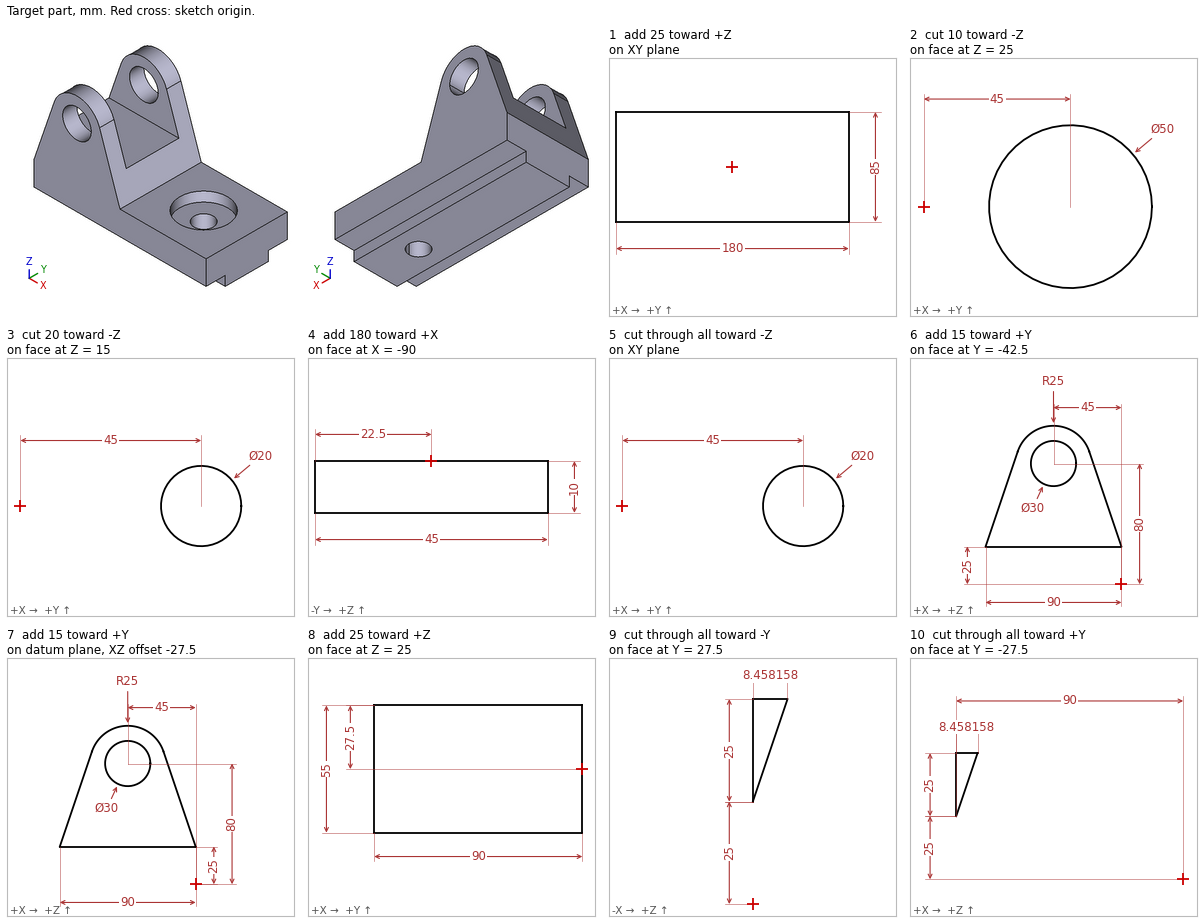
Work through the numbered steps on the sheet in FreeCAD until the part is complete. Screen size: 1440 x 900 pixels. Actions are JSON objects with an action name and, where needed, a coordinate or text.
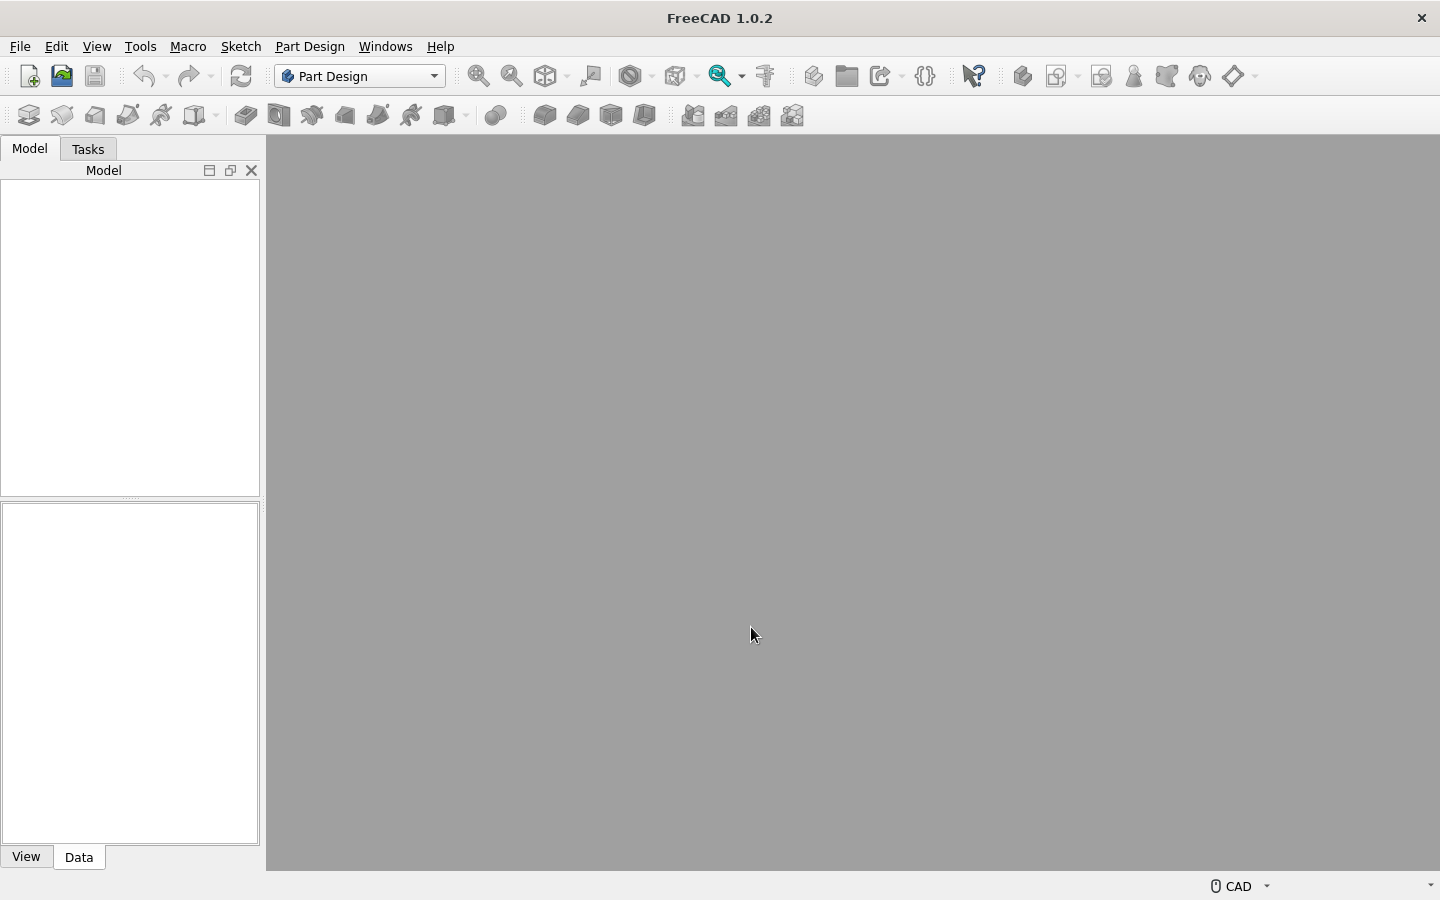
{"action": "left_click", "coordinate": [29, 76]}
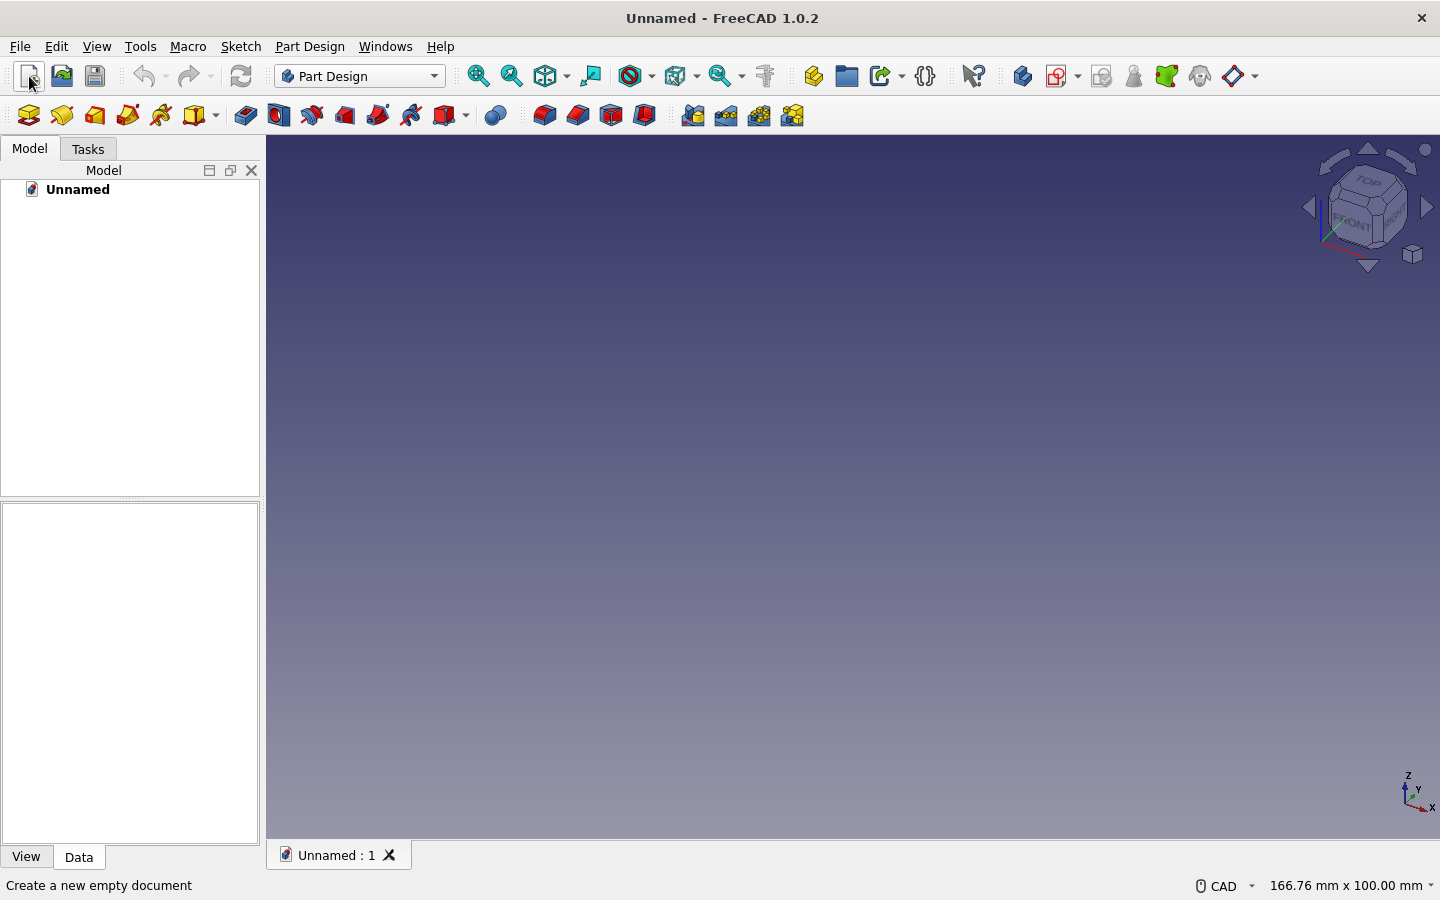
{"action": "left_click", "coordinate": [1056, 76]}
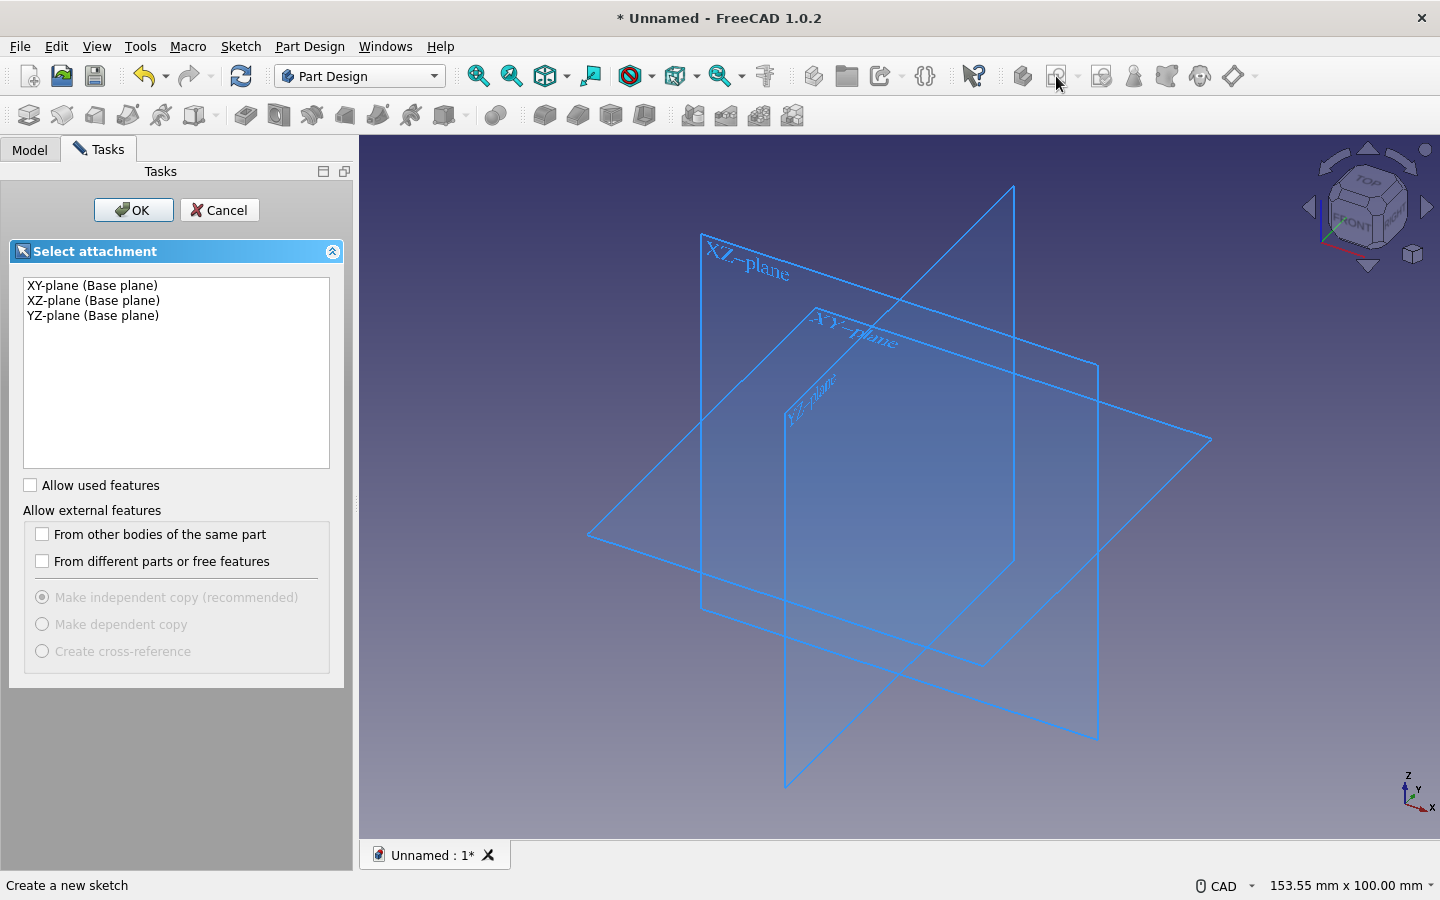
{"action": "left_click", "coordinate": [84, 286]}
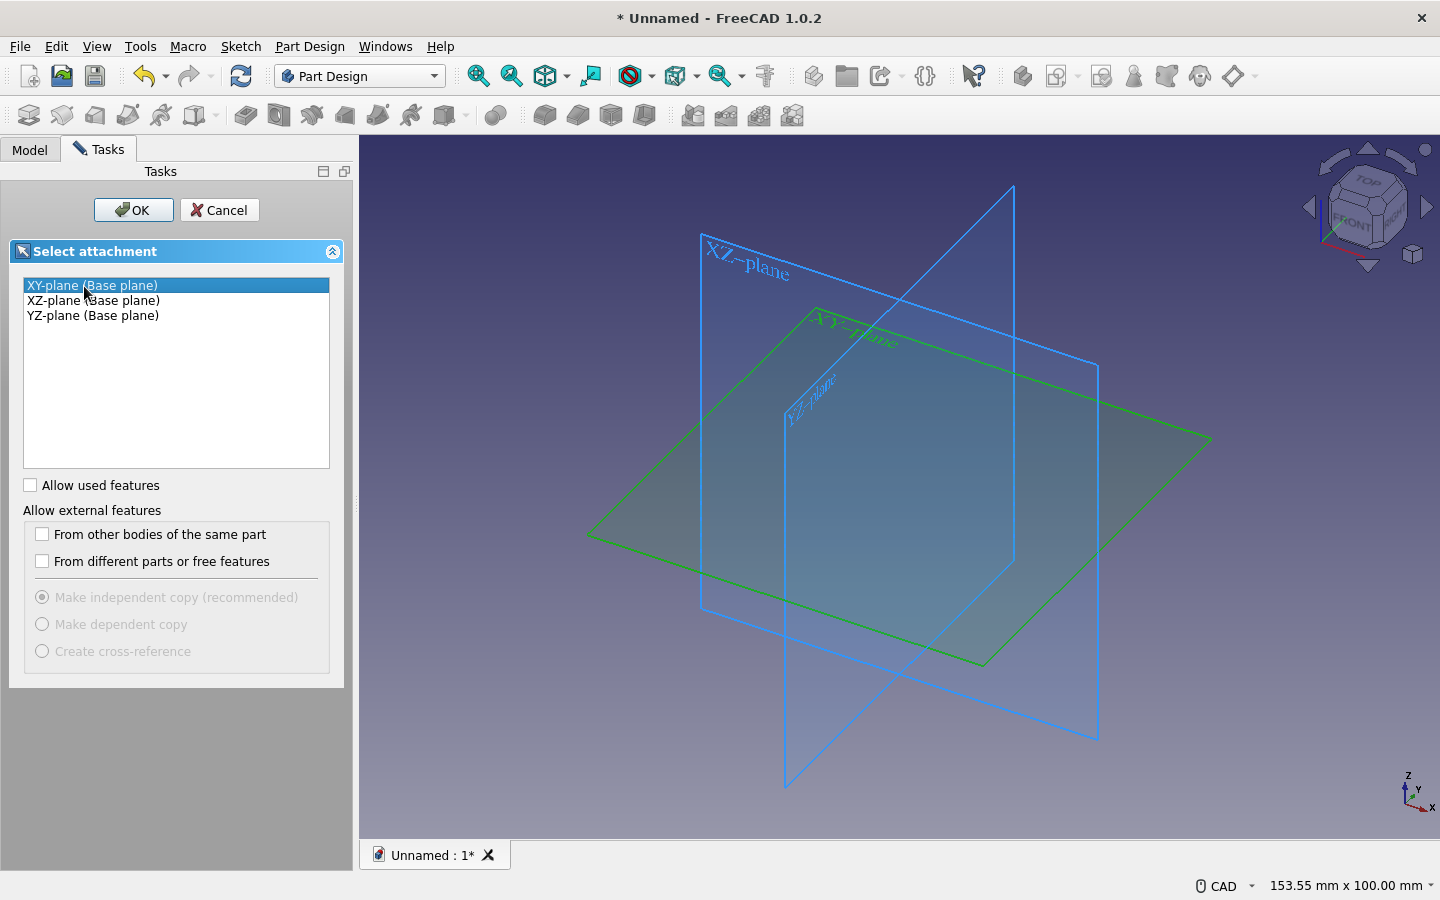
{"action": "left_click", "coordinate": [134, 210]}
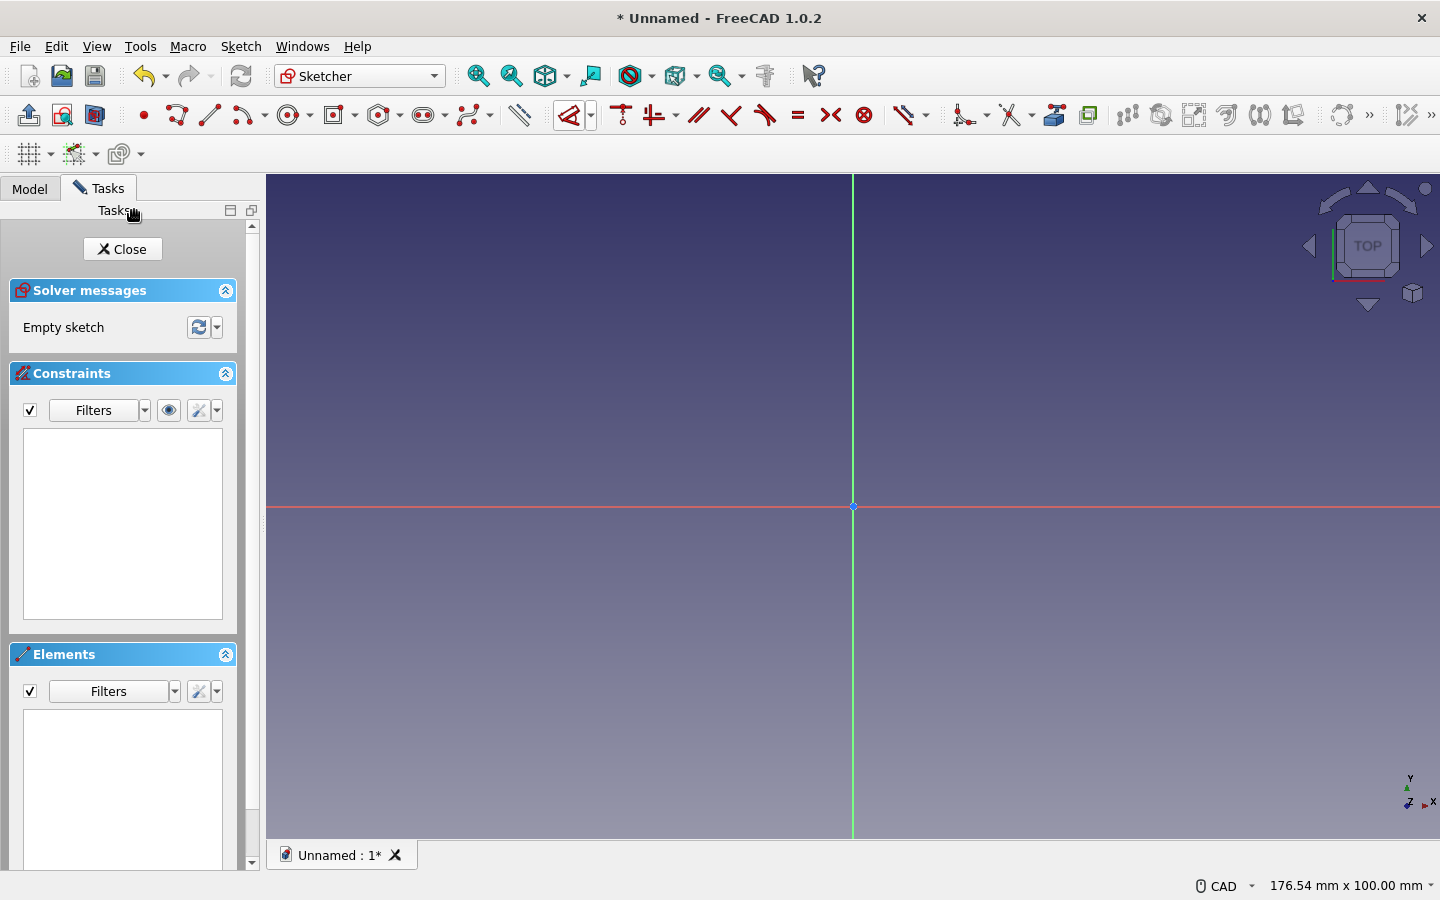
{"action": "scroll", "coordinate": [701, 506], "scroll_direction": "down", "scroll_amount": 3}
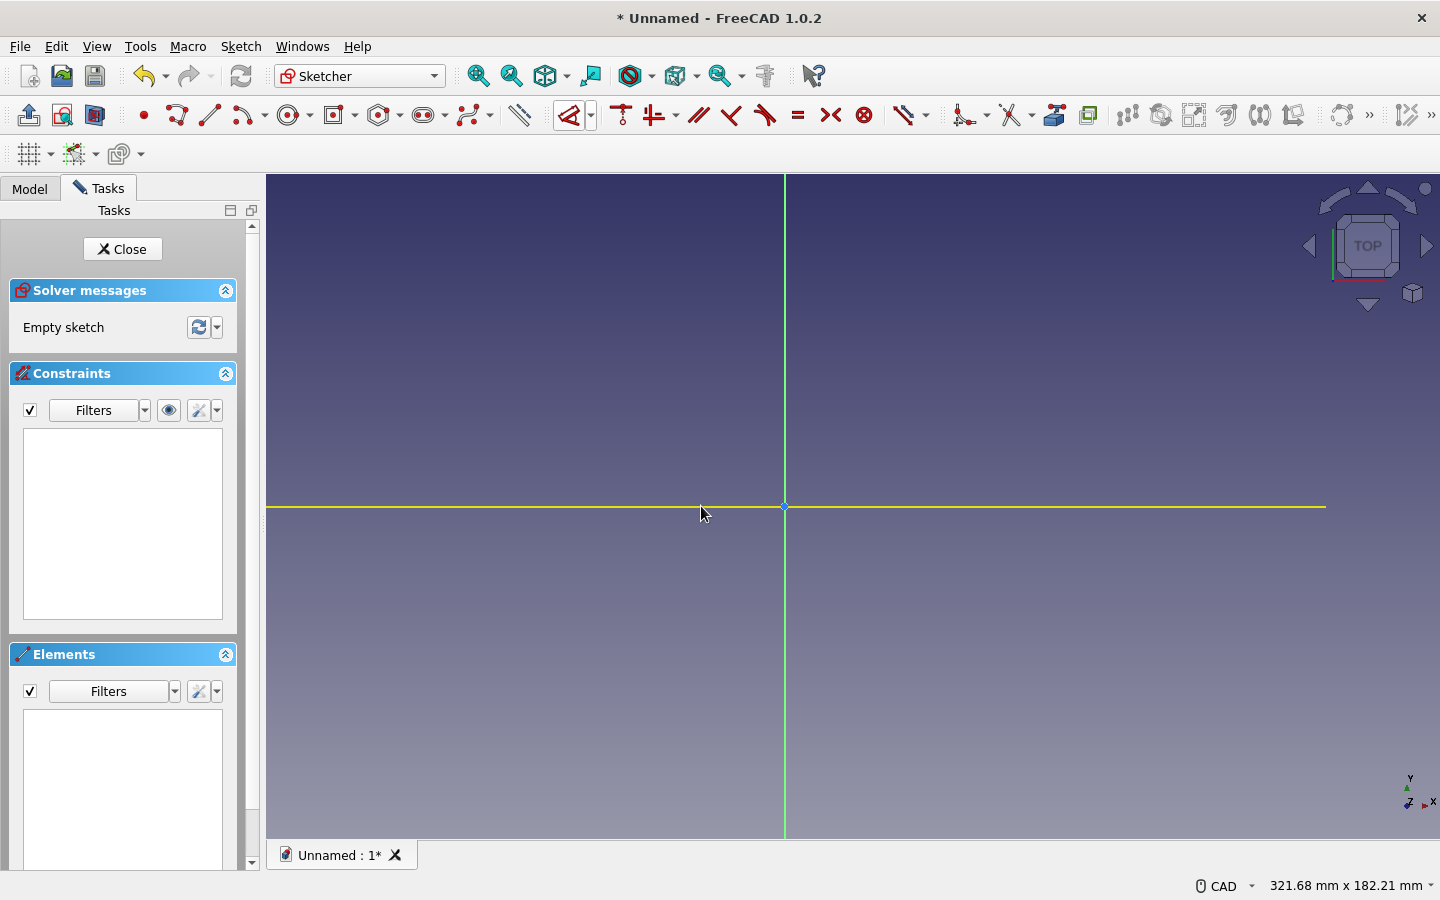
{"action": "left_click", "coordinate": [332, 116]}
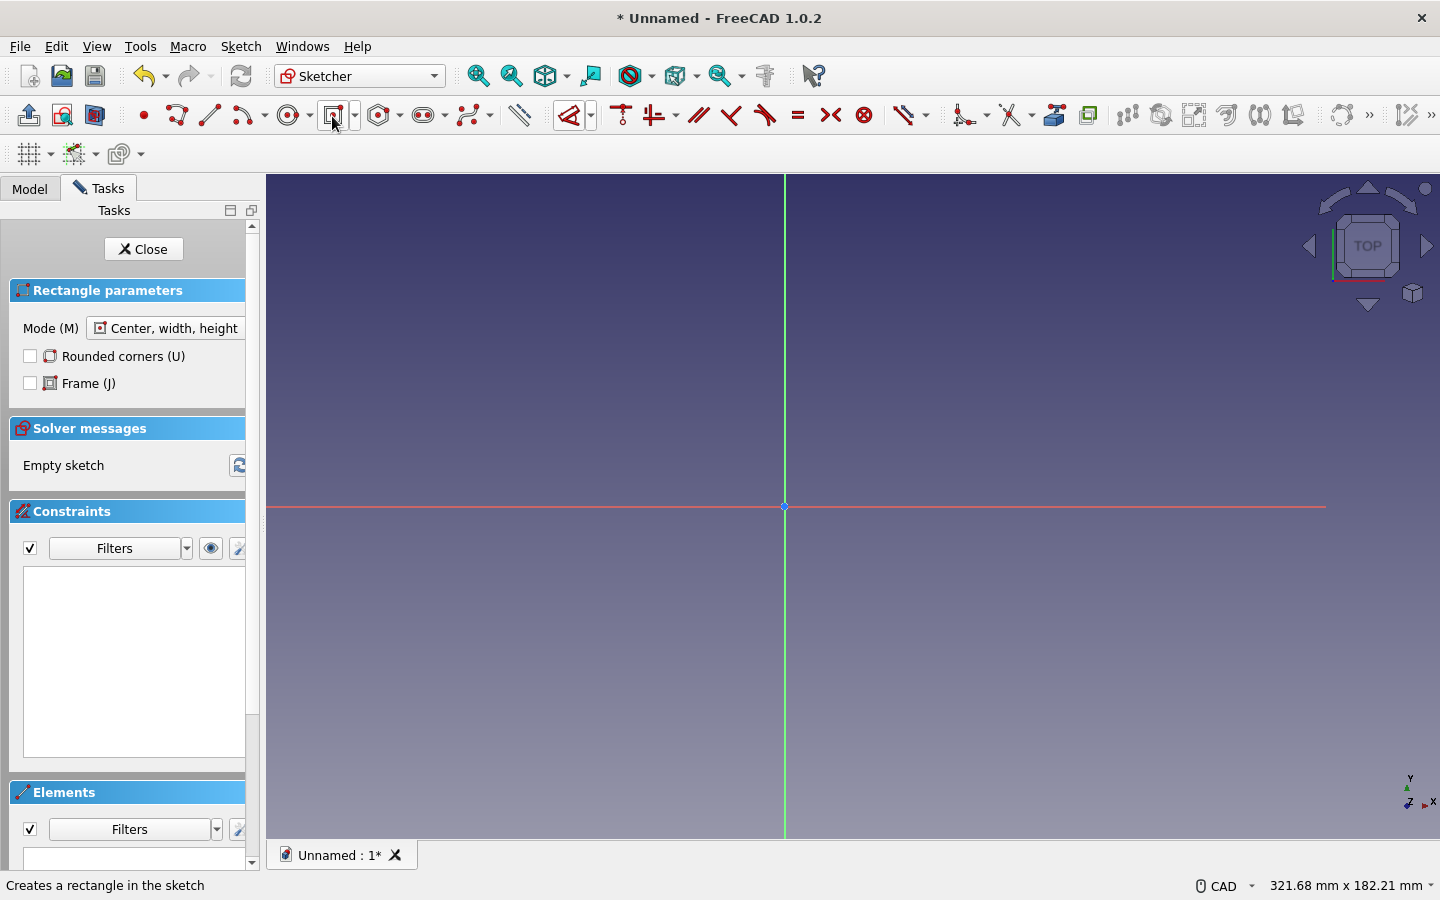
{"action": "left_click", "coordinate": [785, 506]}
{"action": "mouse_move", "coordinate": [1113, 351]}